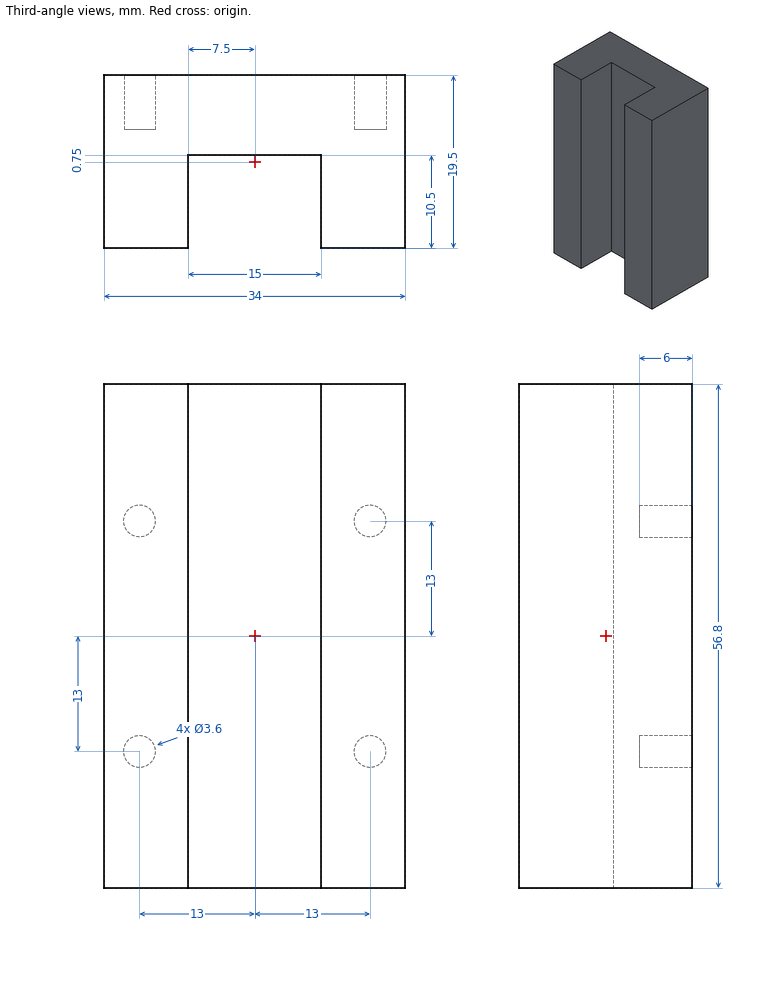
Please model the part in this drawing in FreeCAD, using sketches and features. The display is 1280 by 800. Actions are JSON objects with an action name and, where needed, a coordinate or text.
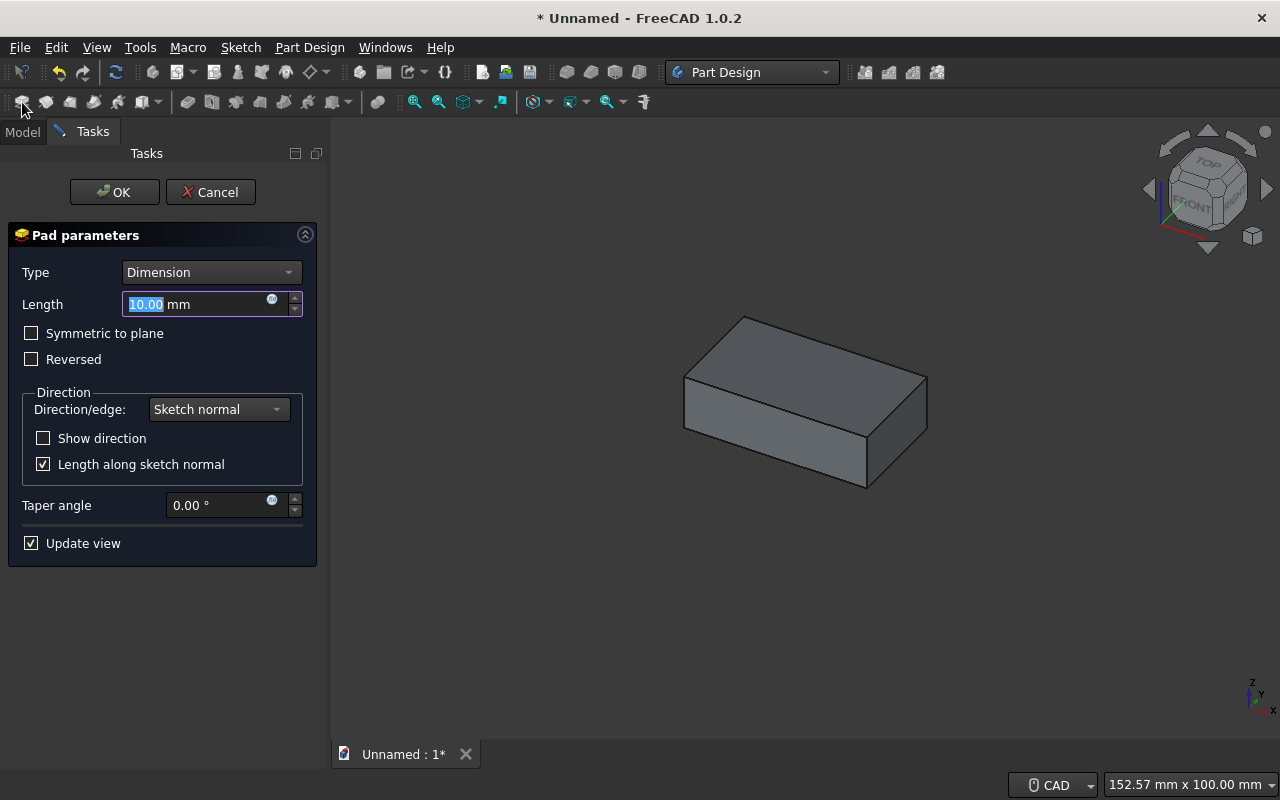
{"action": "type", "text": "56.8"}
{"action": "key", "text": "Tab"}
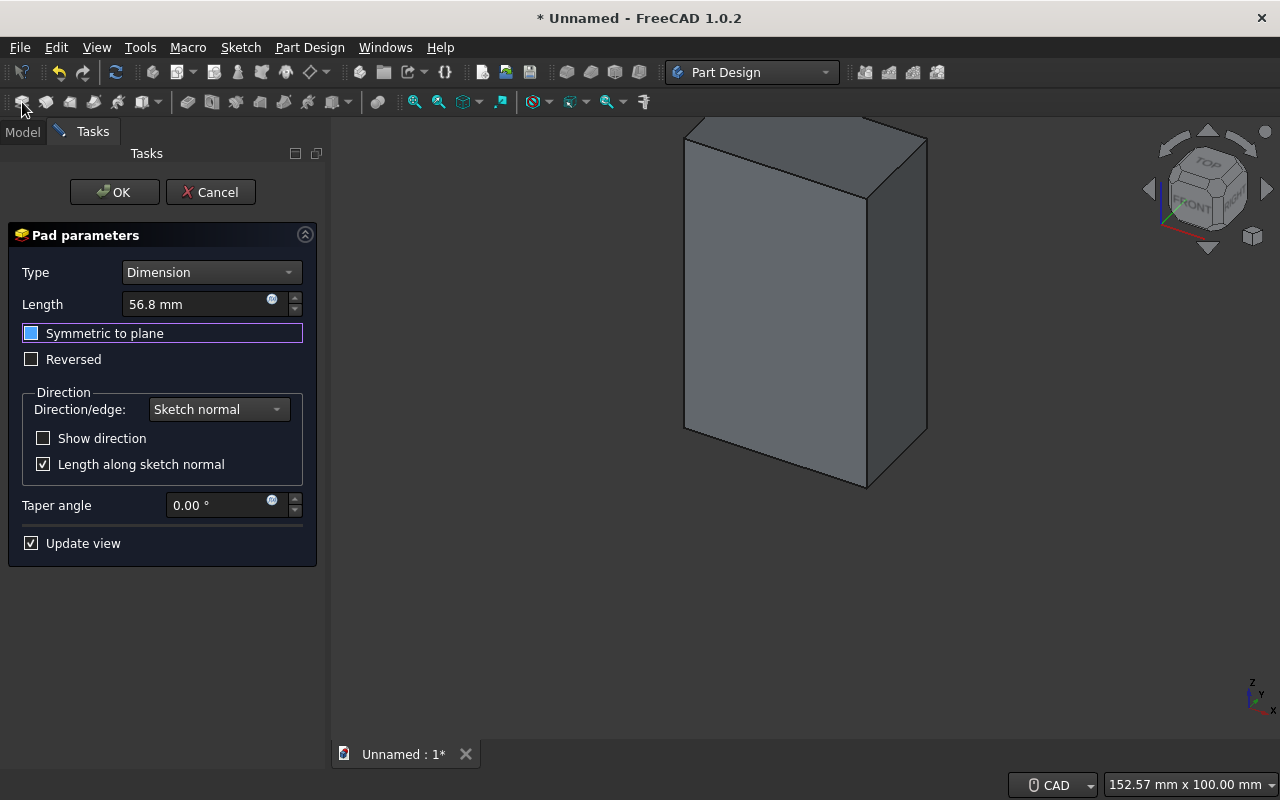
{"action": "left_click", "coordinate": [30, 333]}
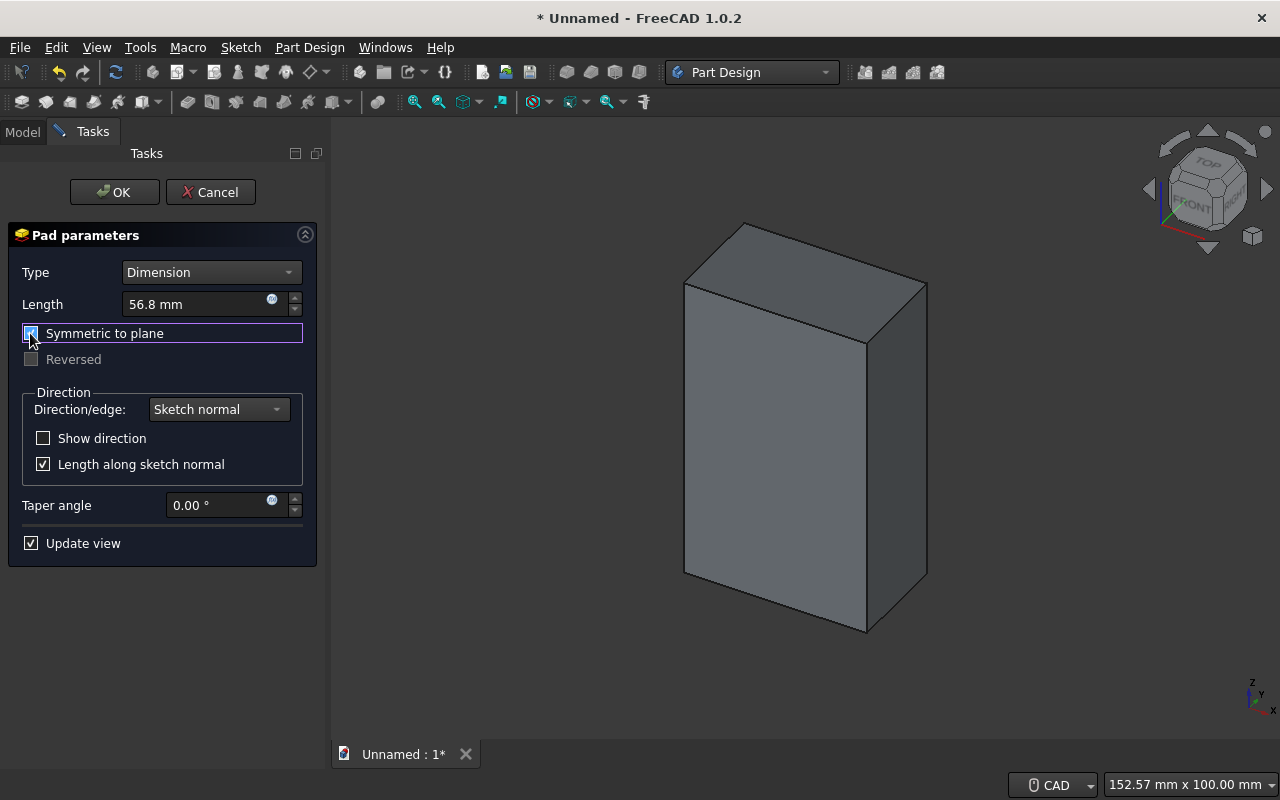
{"action": "left_click", "coordinate": [115, 192]}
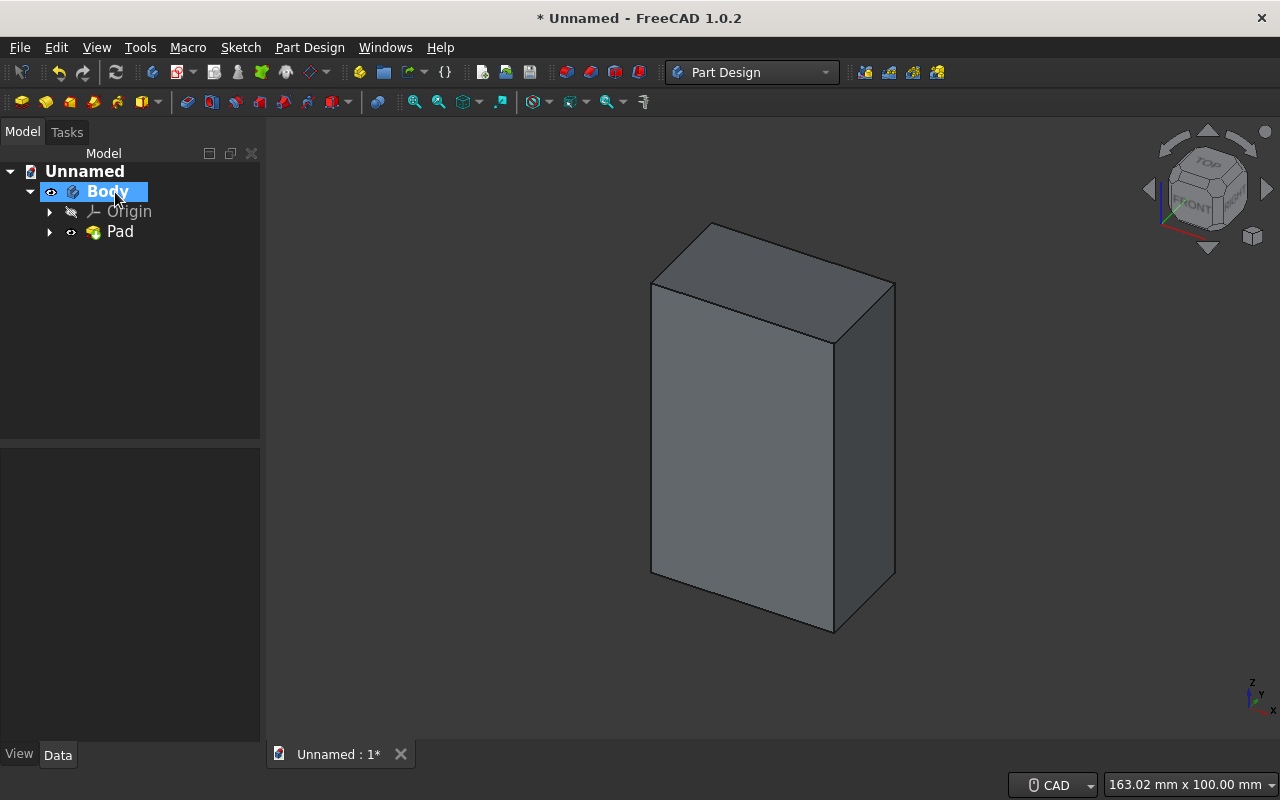
{"action": "left_click", "coordinate": [178, 72]}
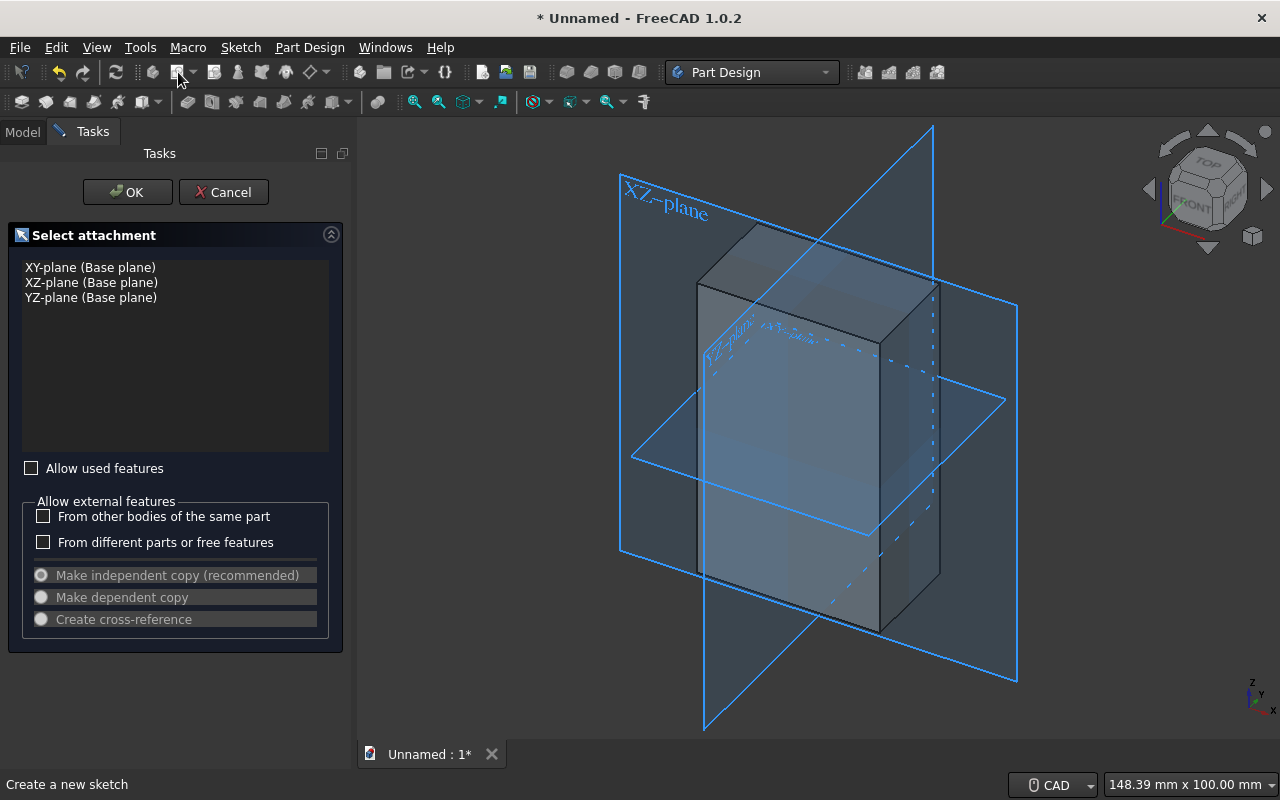
{"action": "left_click", "coordinate": [82, 268]}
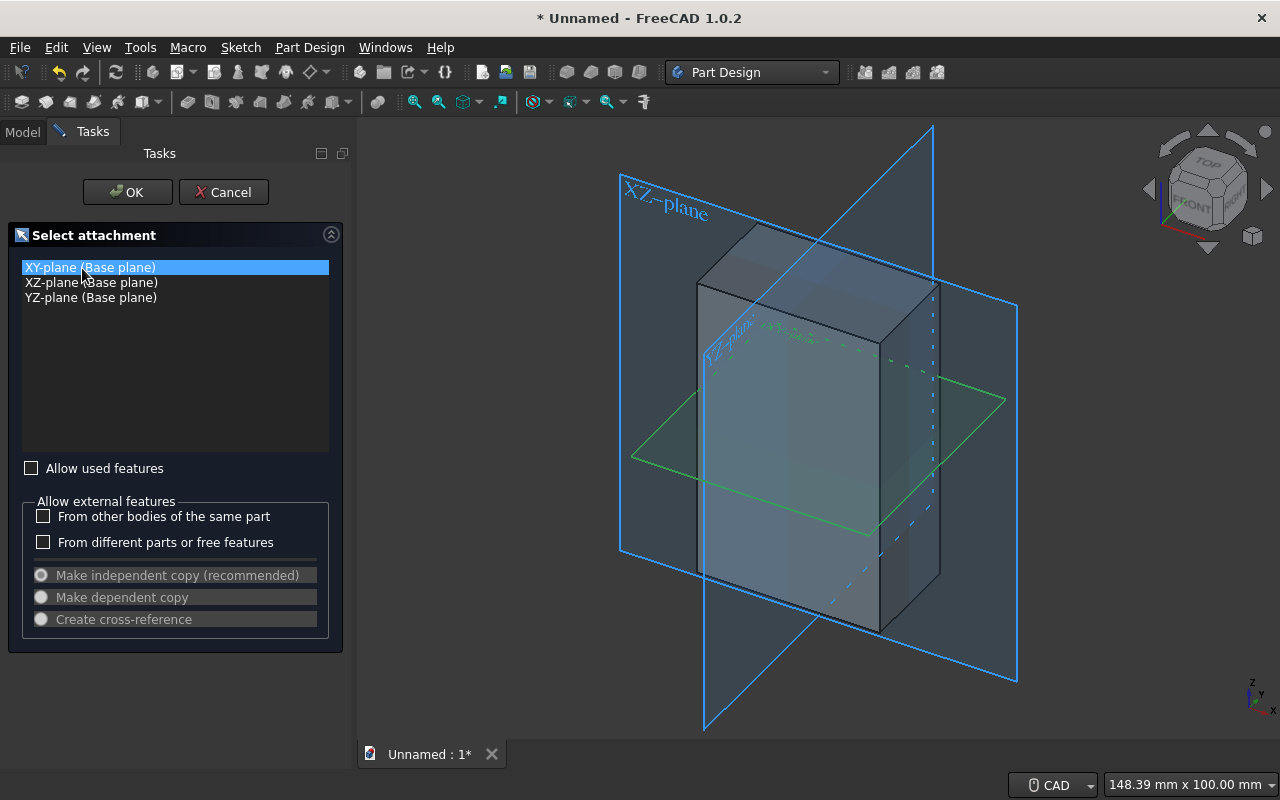
{"action": "left_click", "coordinate": [128, 192]}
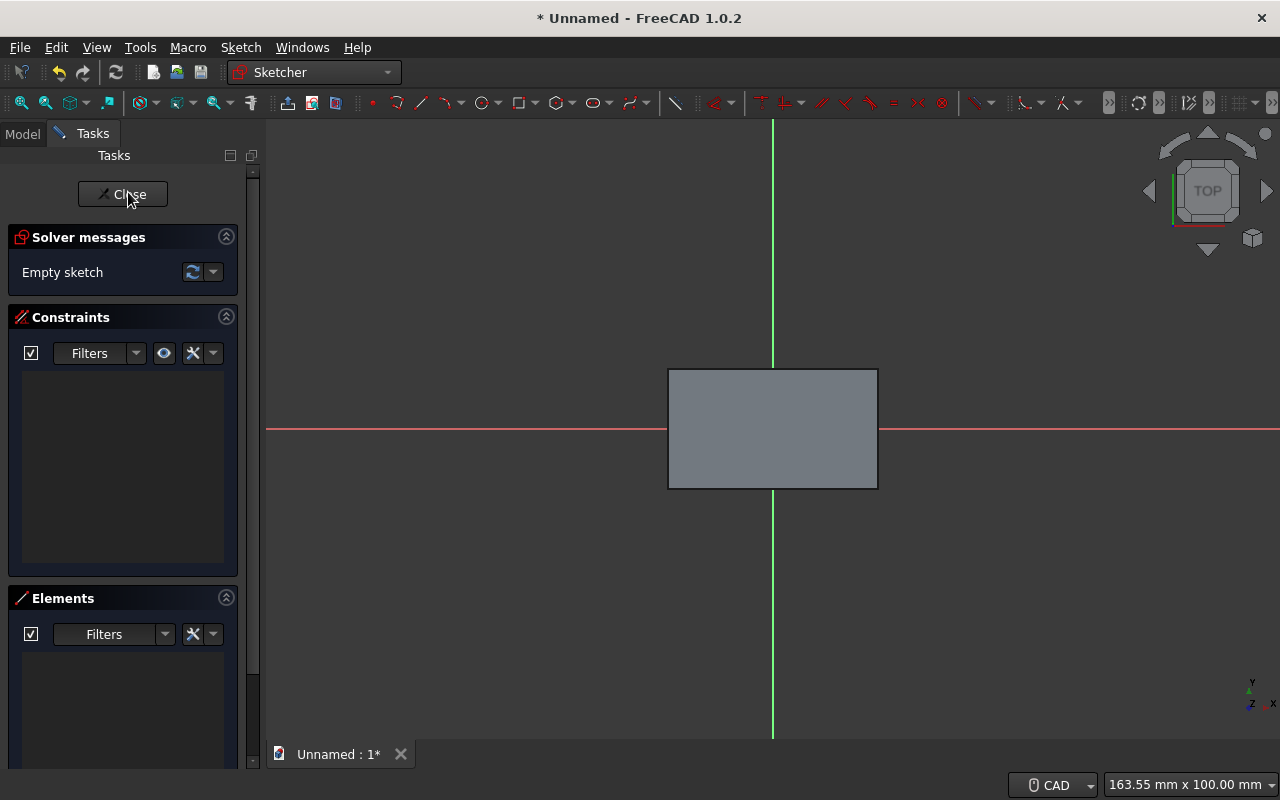
{"action": "left_click", "coordinate": [336, 104]}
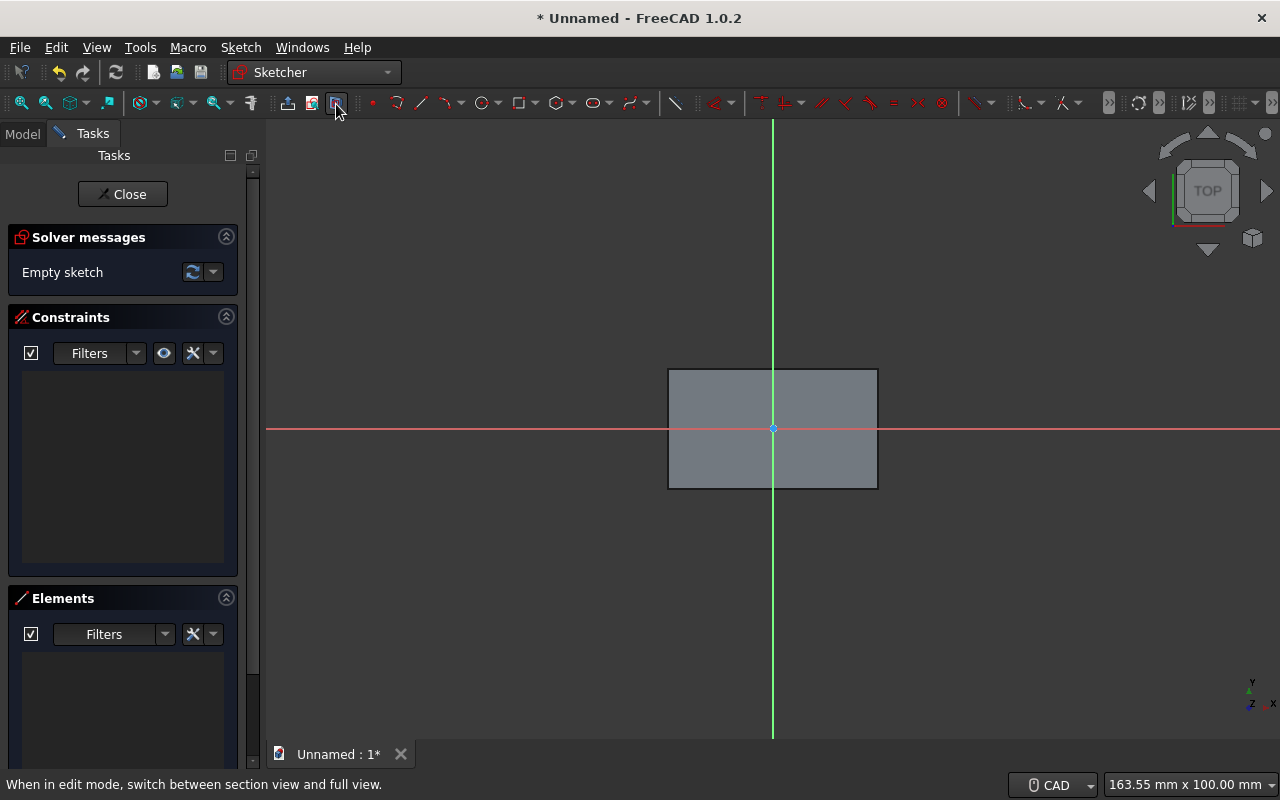
{"action": "scroll", "coordinate": [787, 462], "scroll_direction": "up", "scroll_amount": 9}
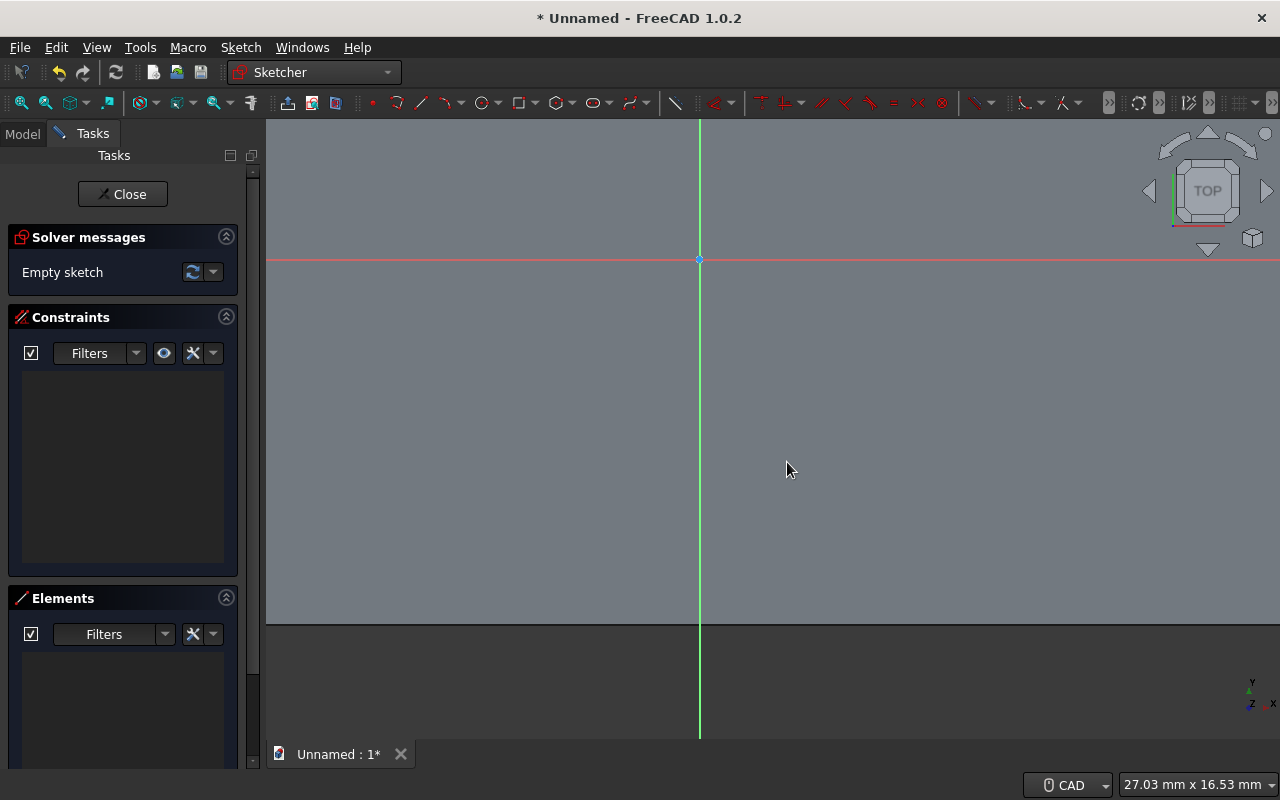
{"action": "left_click", "coordinate": [520, 104]}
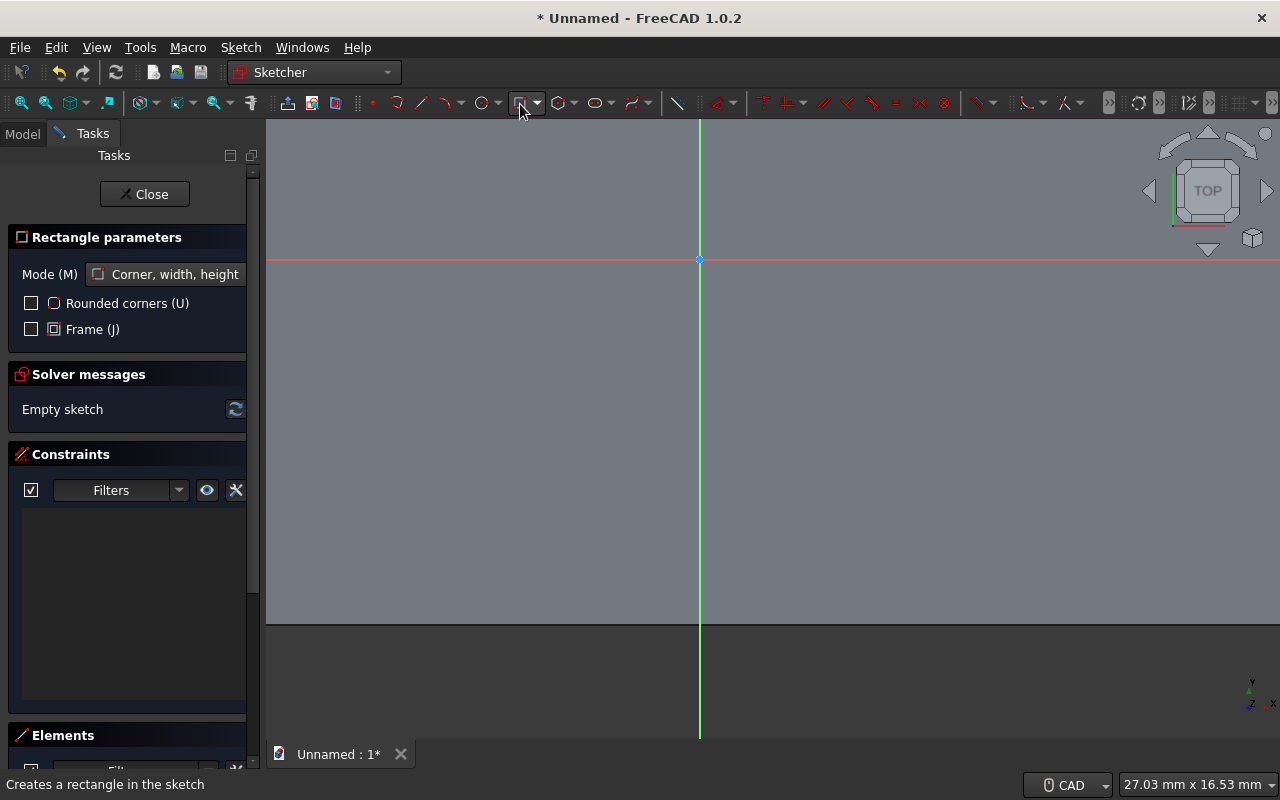
{"action": "left_click", "coordinate": [418, 231]}
{"action": "mouse_move", "coordinate": [981, 625]}